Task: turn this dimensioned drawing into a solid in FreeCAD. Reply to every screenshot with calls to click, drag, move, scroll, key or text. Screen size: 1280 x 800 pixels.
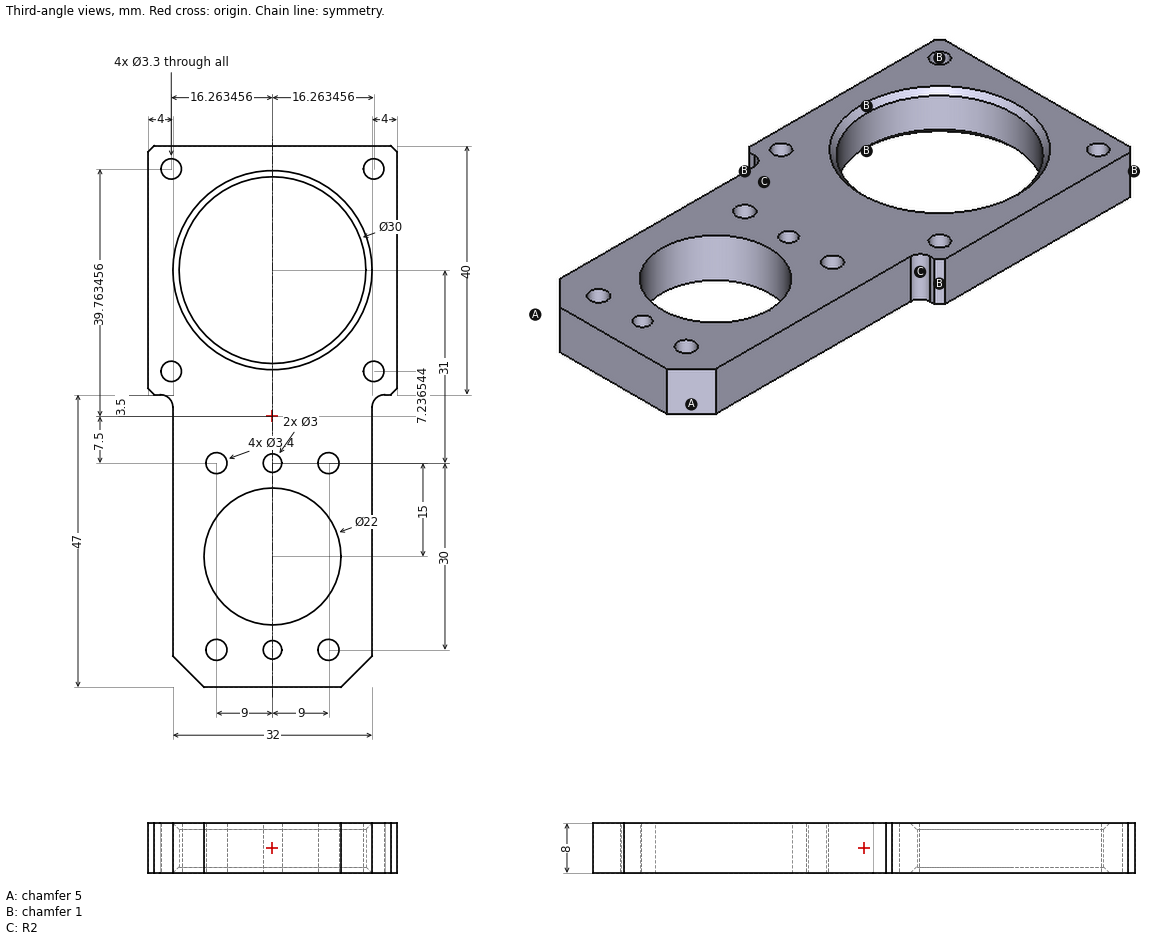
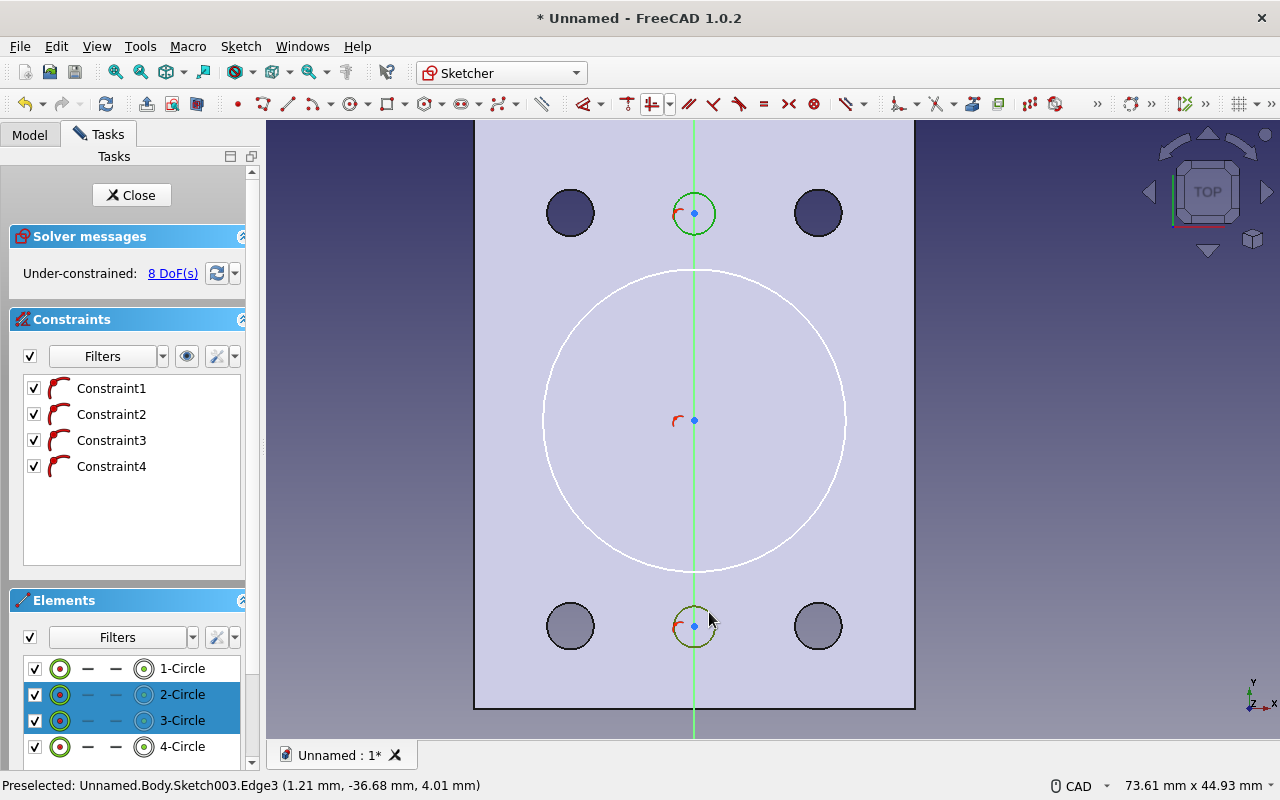
key(e)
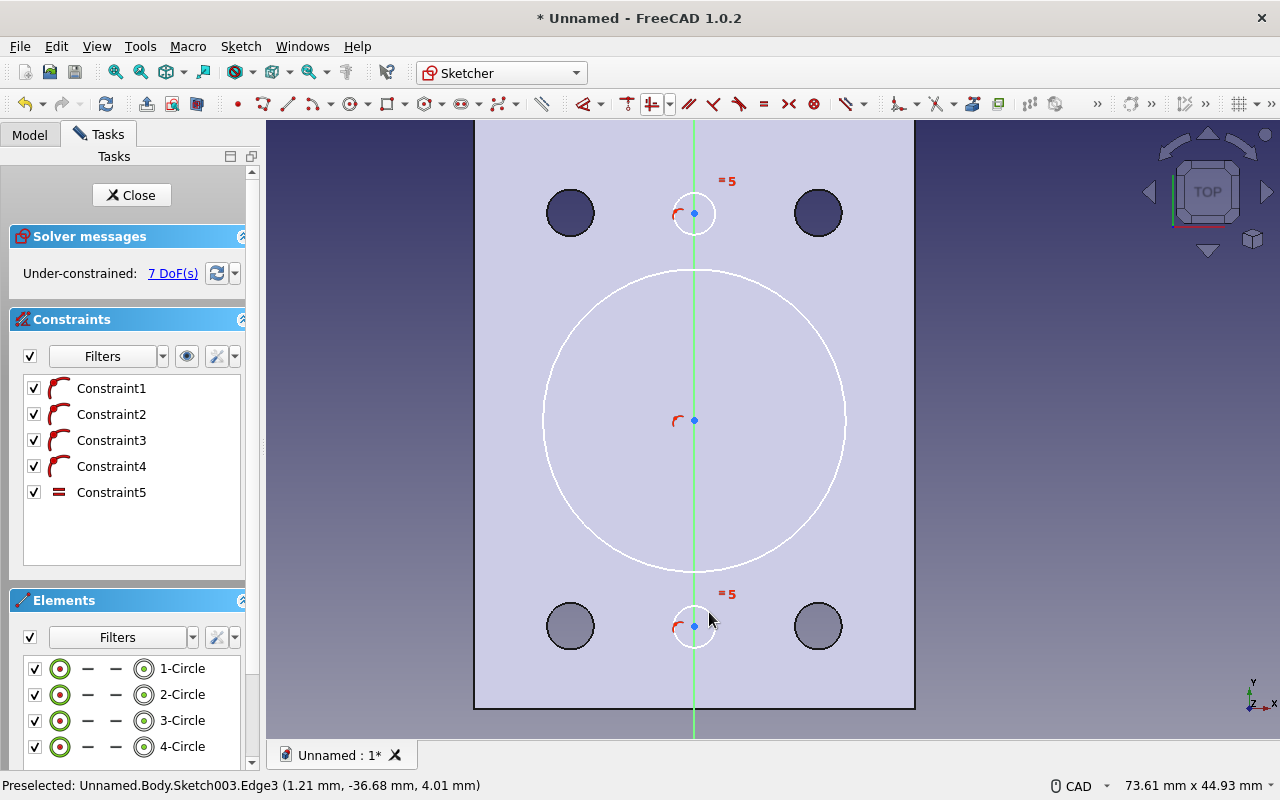
click(582, 104)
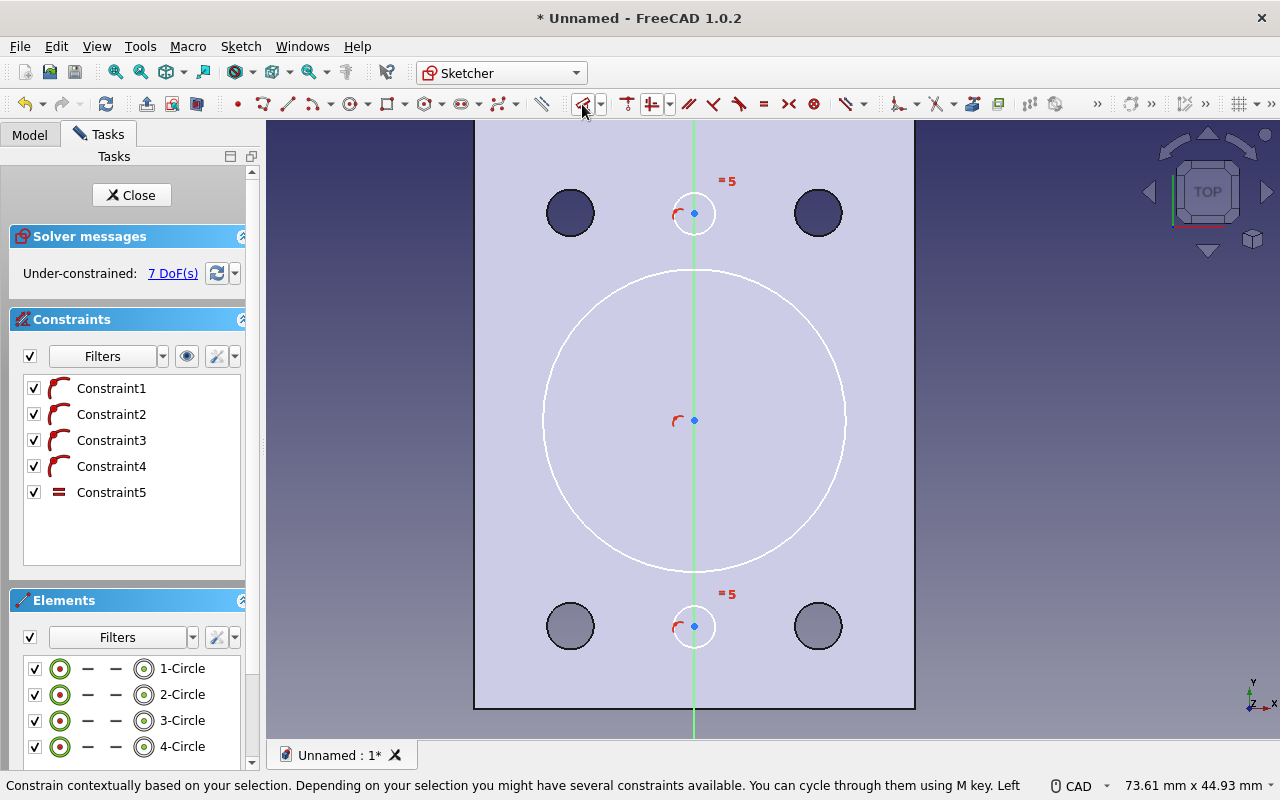
scroll(710, 614, down, 5)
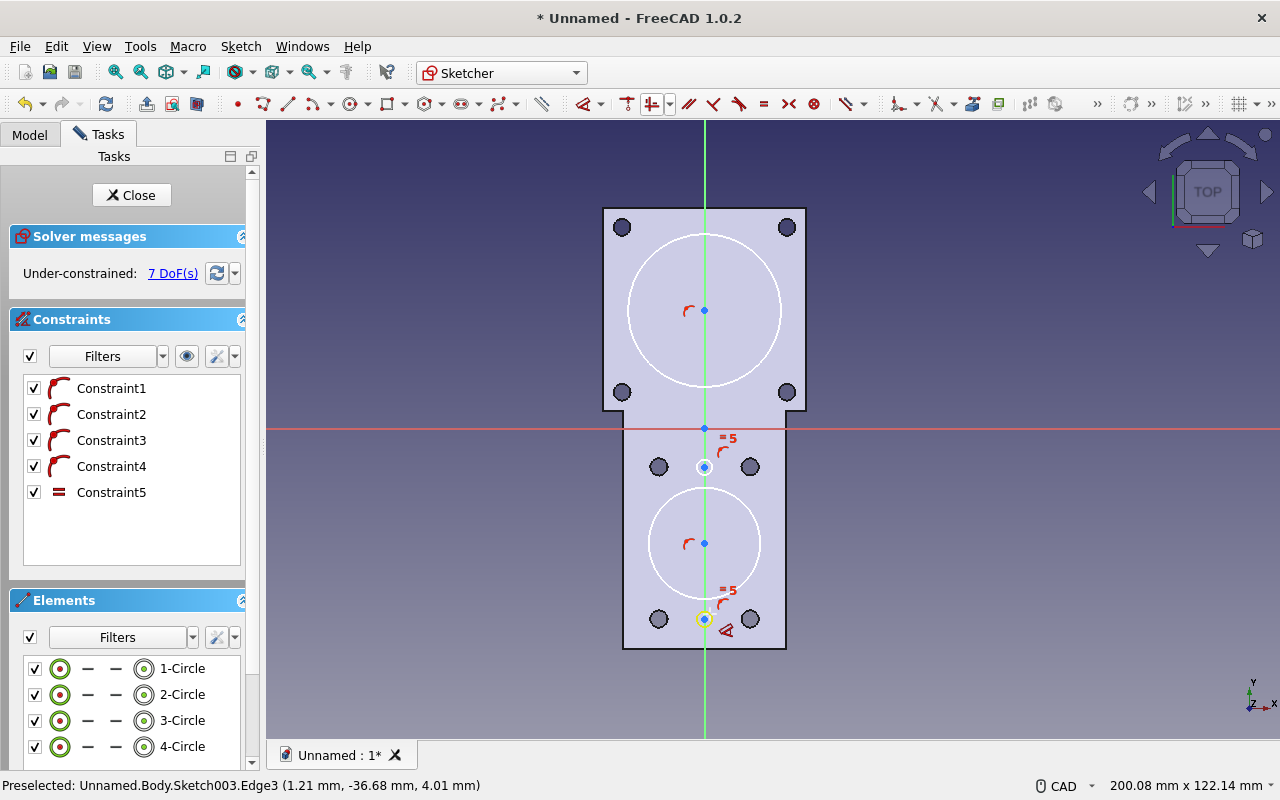
click(758, 256)
click(780, 233)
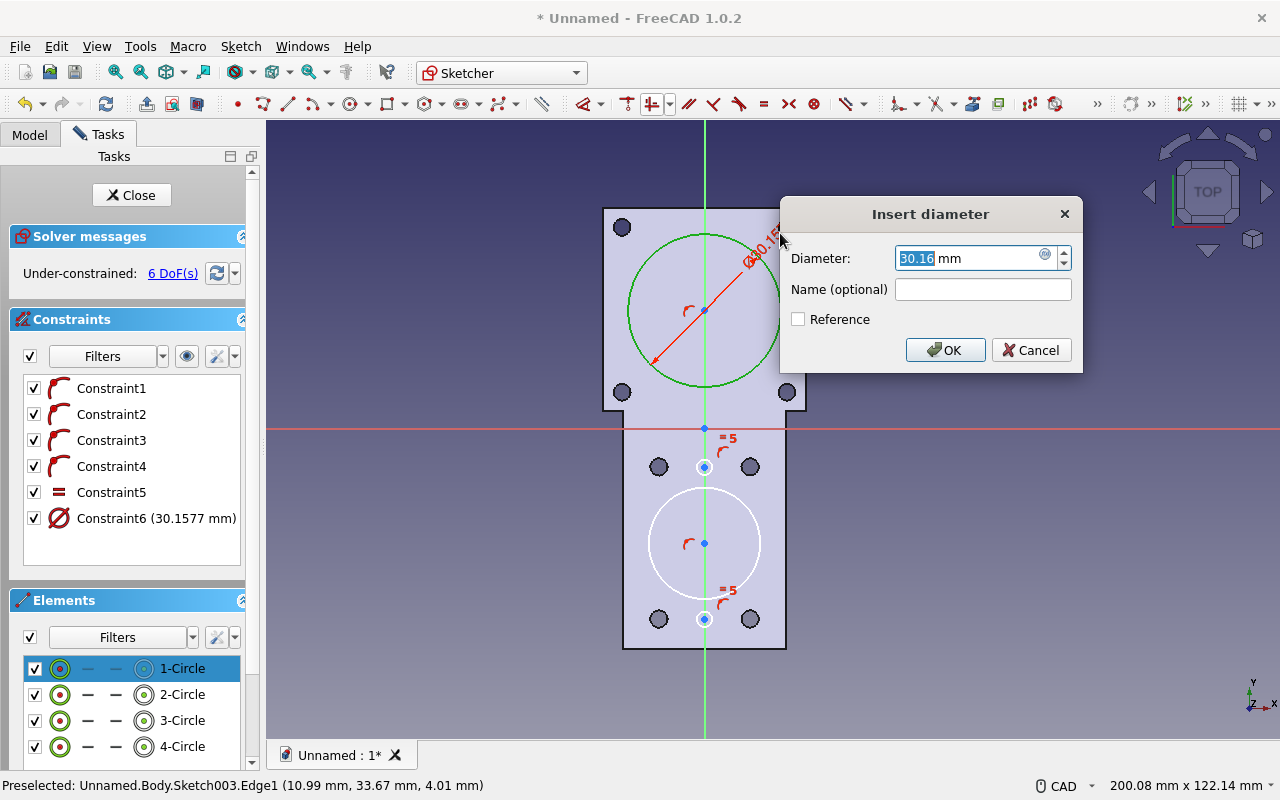
text(30)
key(Return)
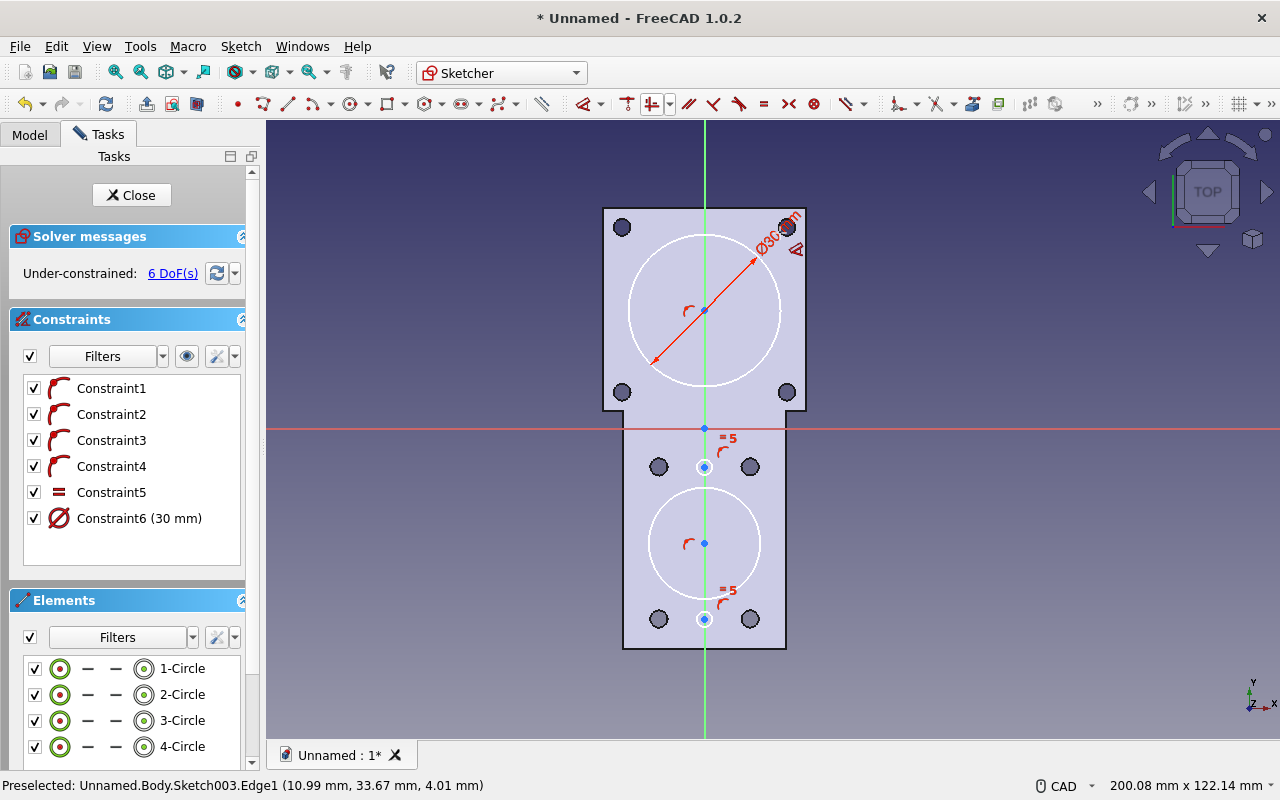
scroll(705, 460, up, 5)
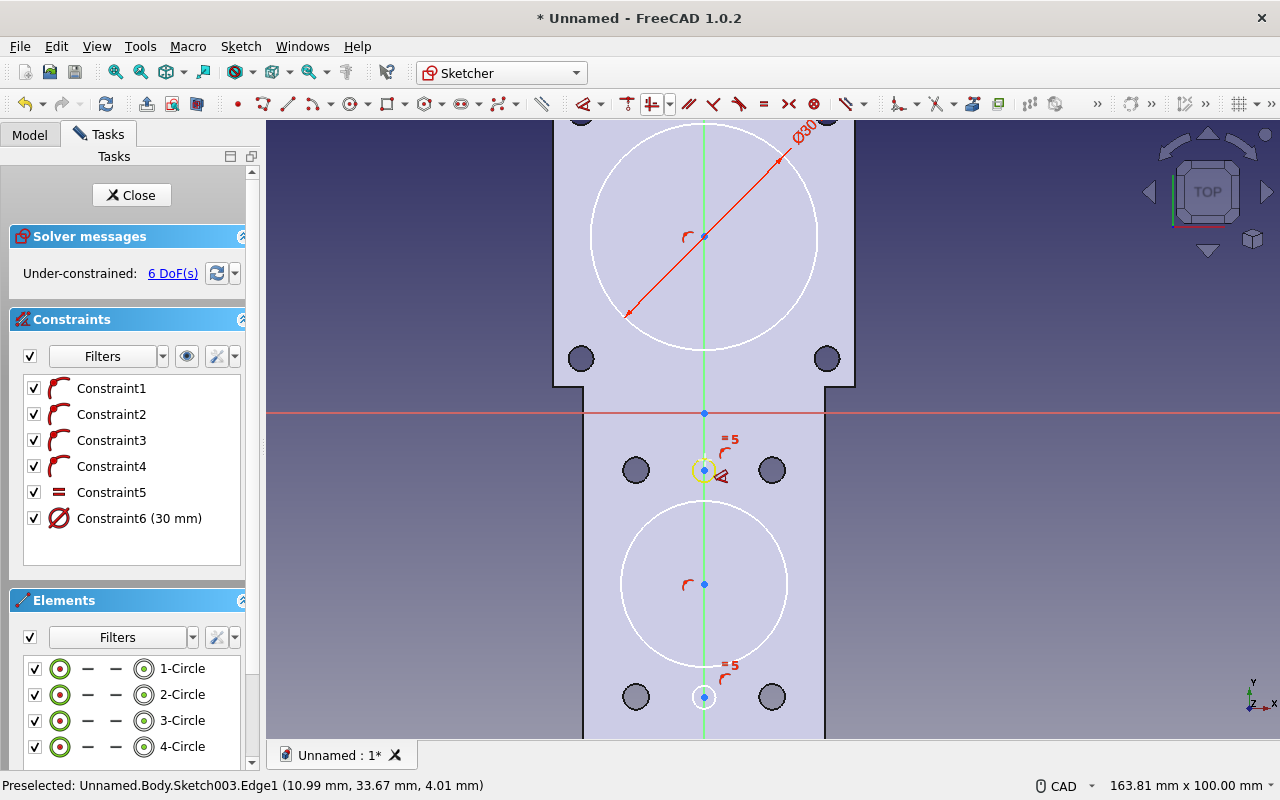
click(704, 458)
click(731, 434)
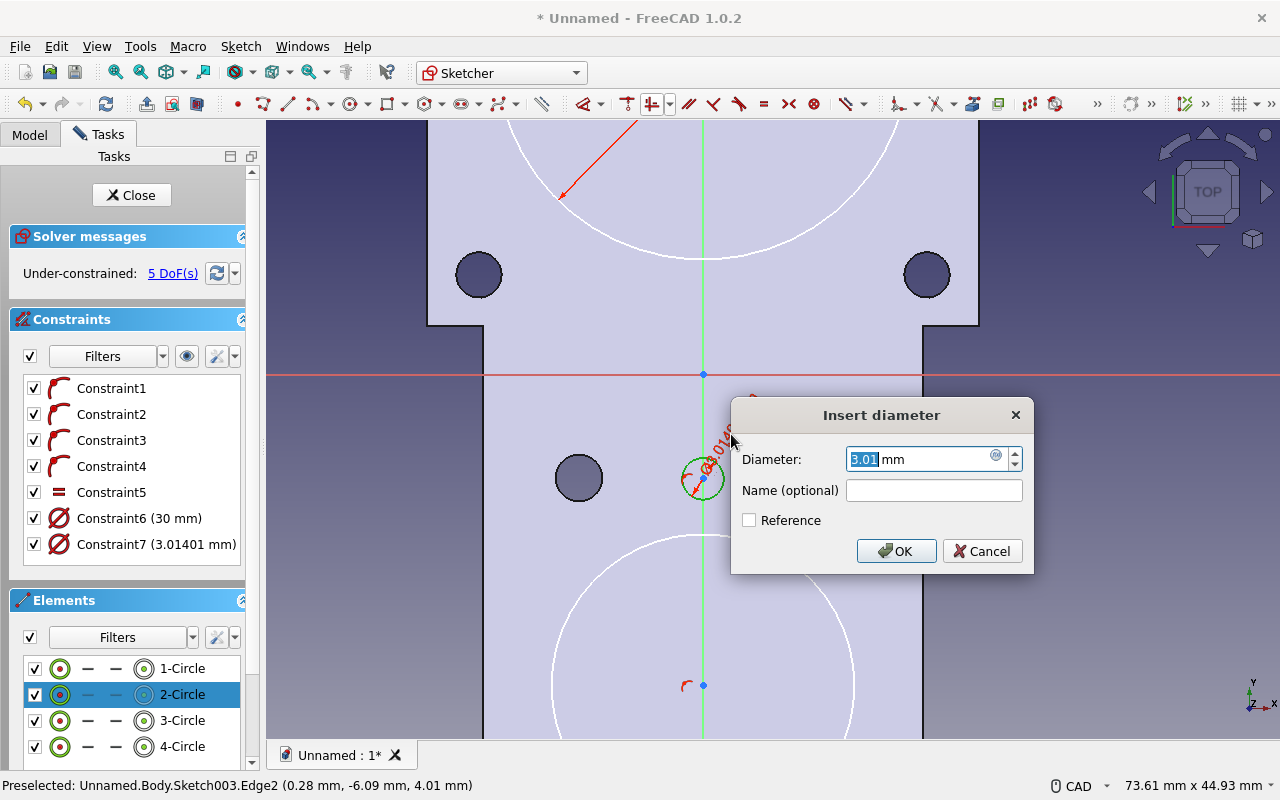
text(3)
key(Return)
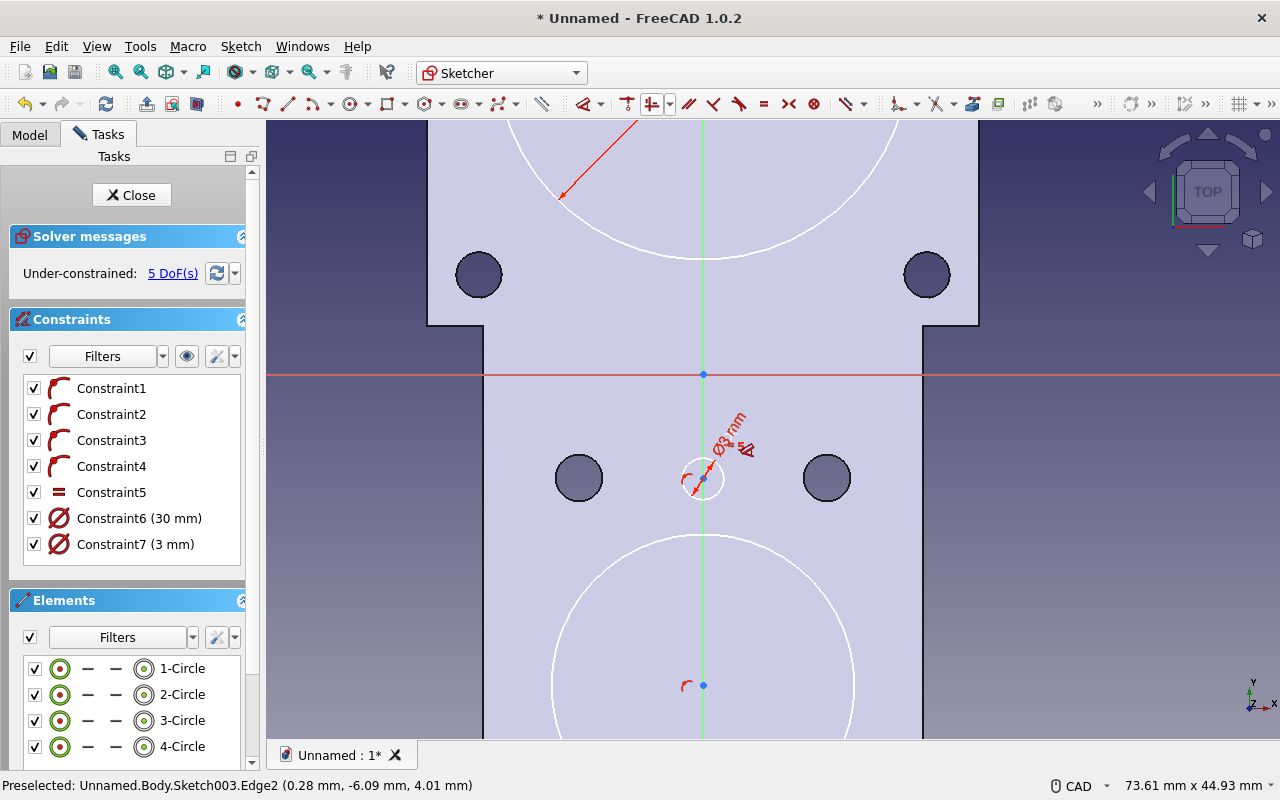
click(810, 578)
click(833, 555)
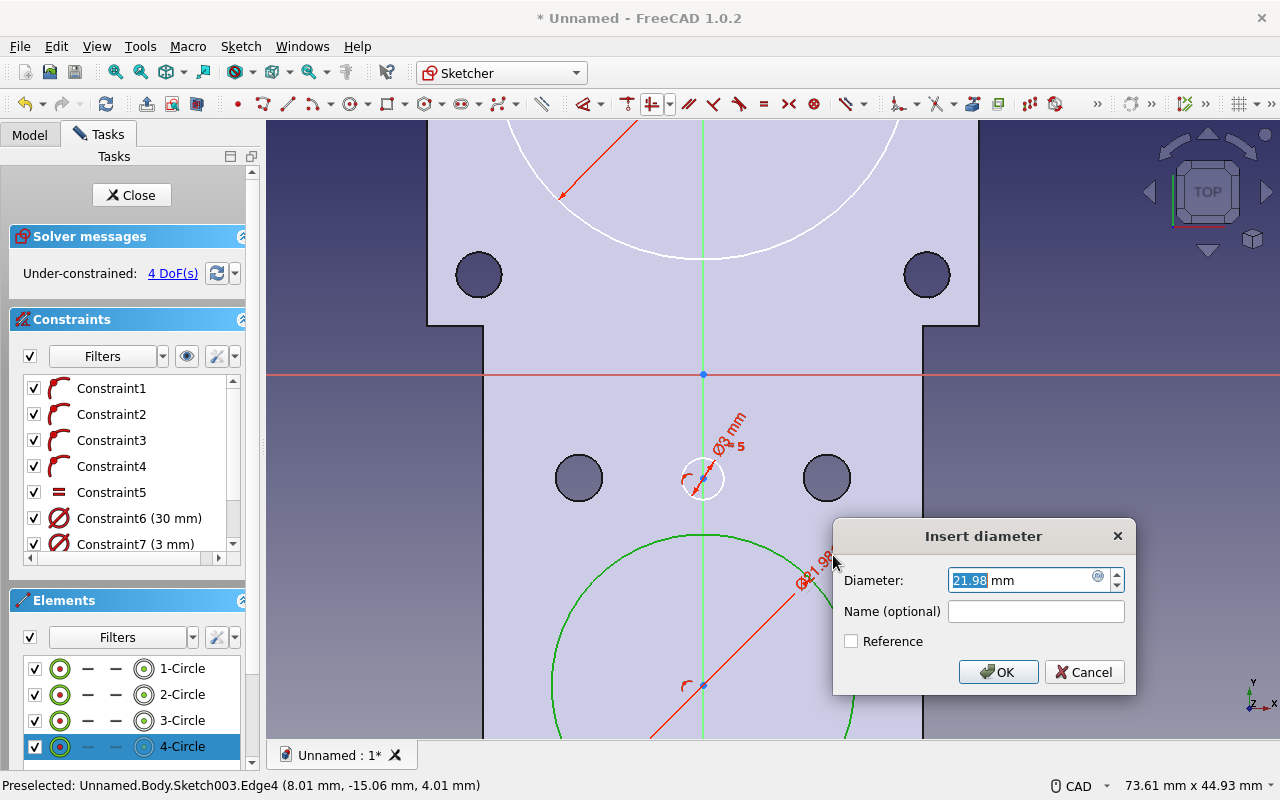
text(22)
key(Return)